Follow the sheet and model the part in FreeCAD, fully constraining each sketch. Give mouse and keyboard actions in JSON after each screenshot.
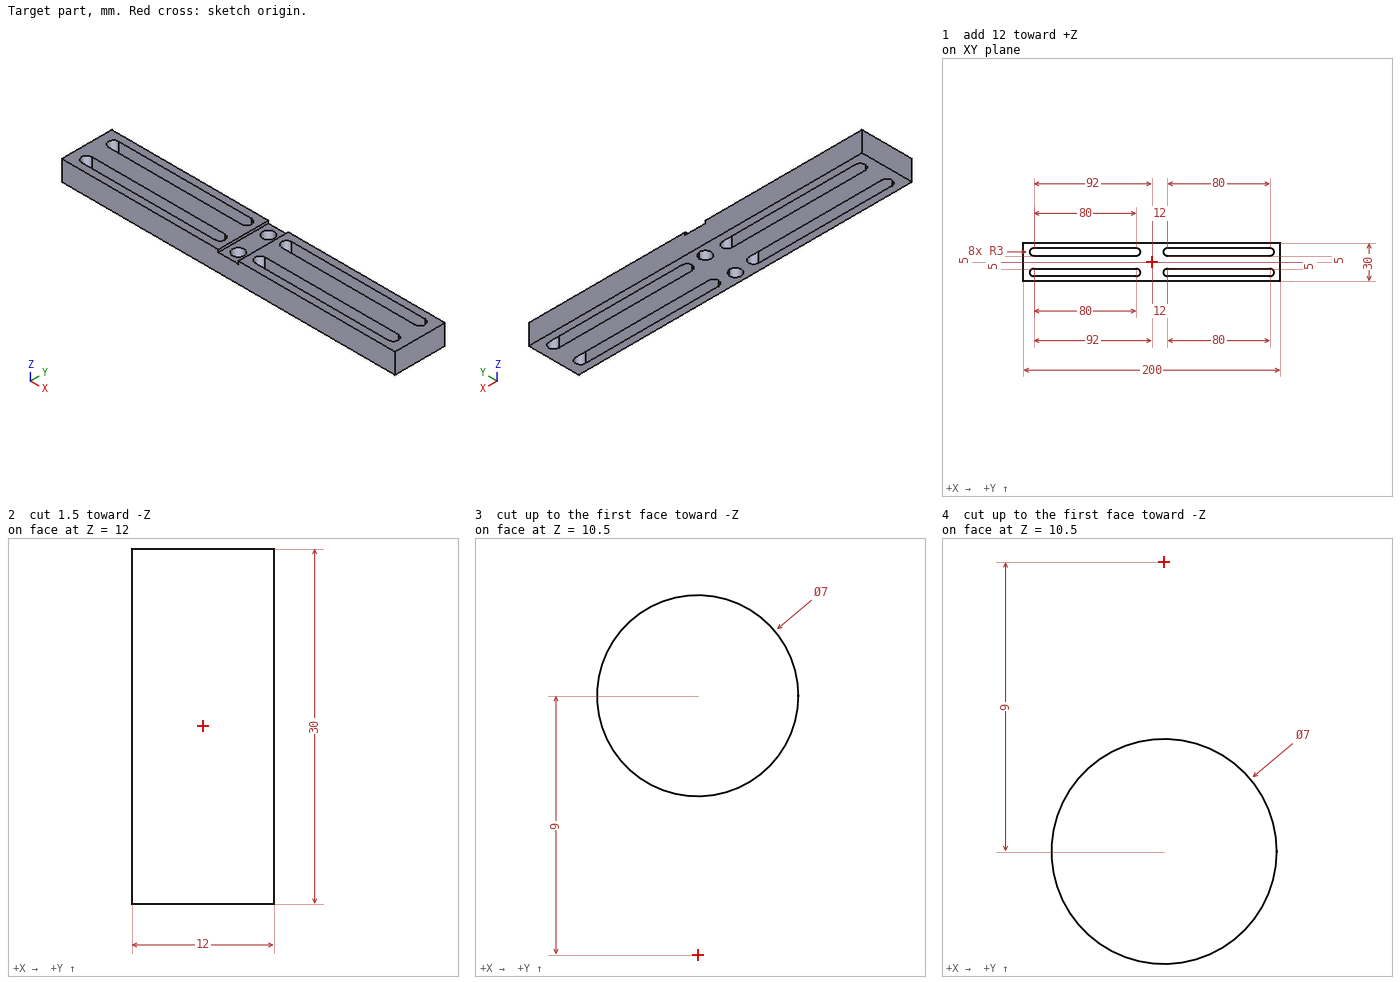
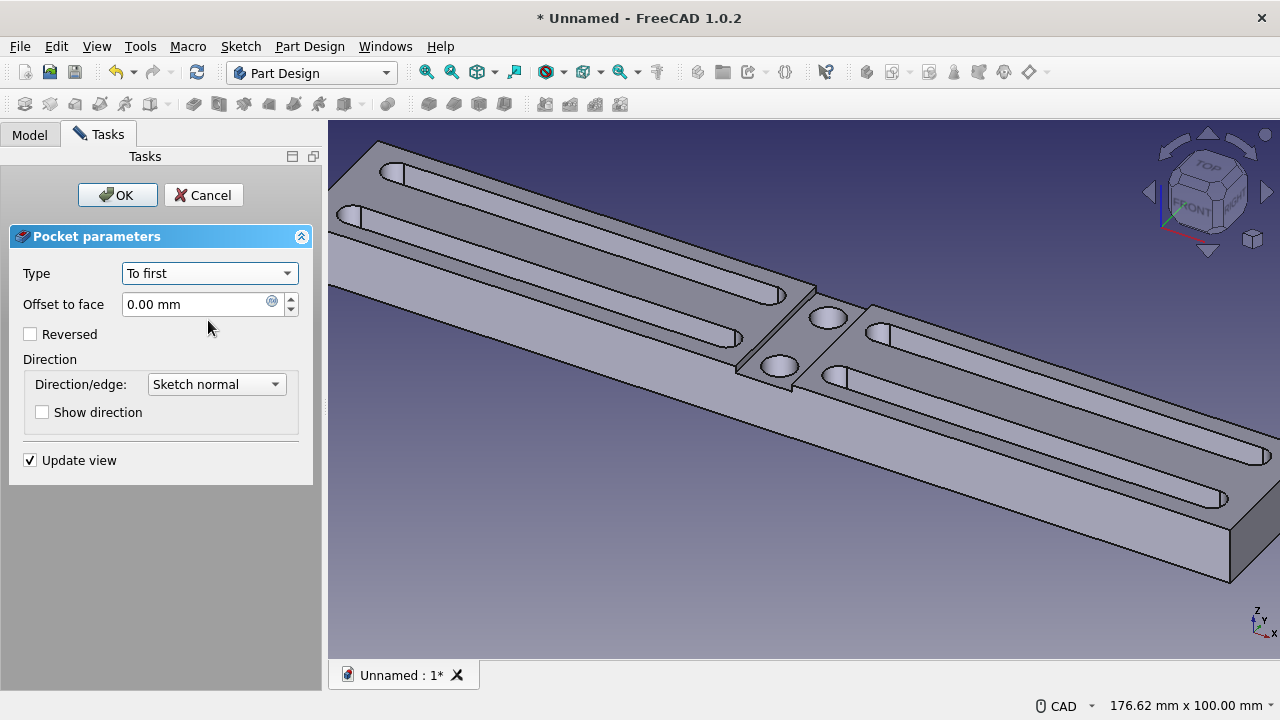
{"action": "left_click", "coordinate": [118, 195]}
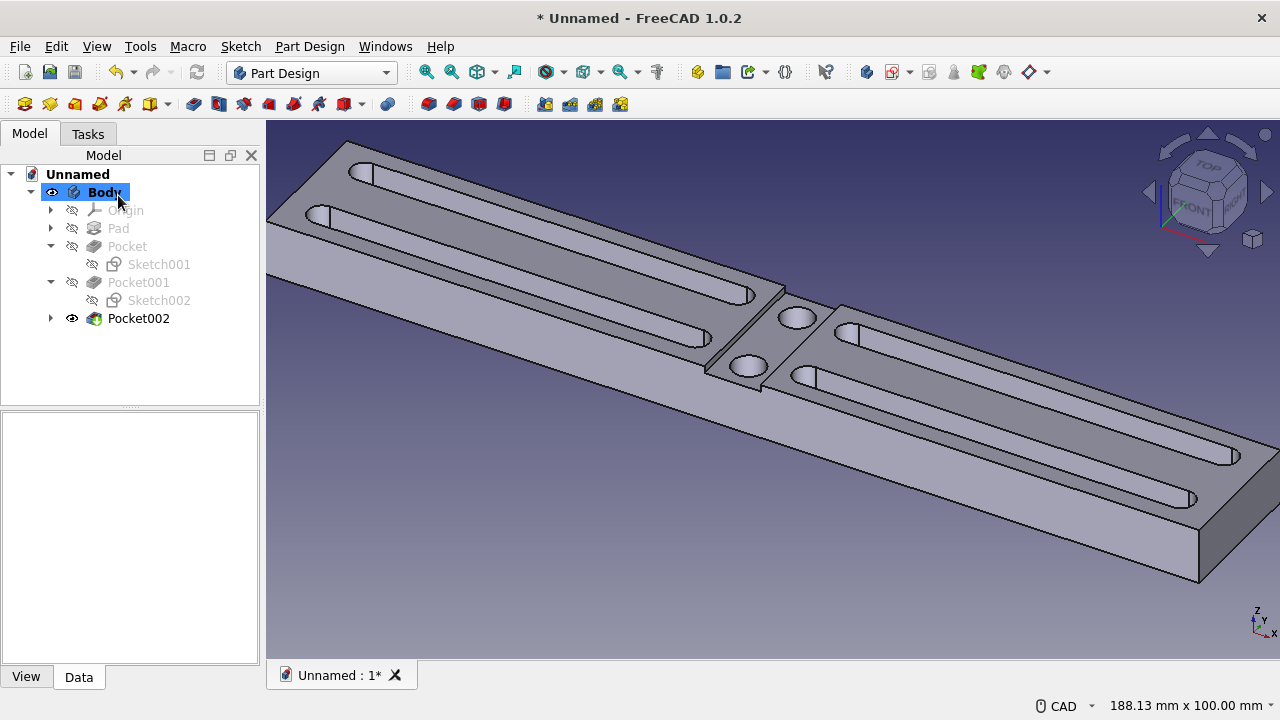
{"action": "key", "text": "0"}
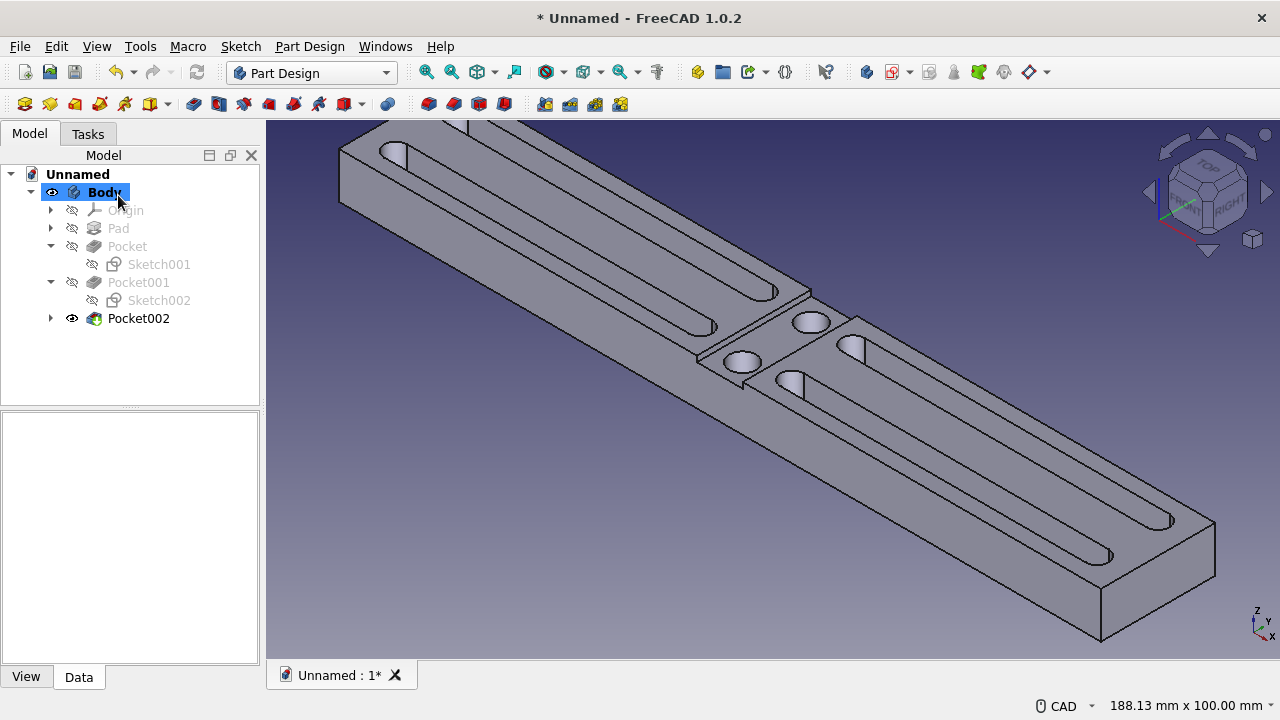
{"action": "left_click", "coordinate": [427, 72]}